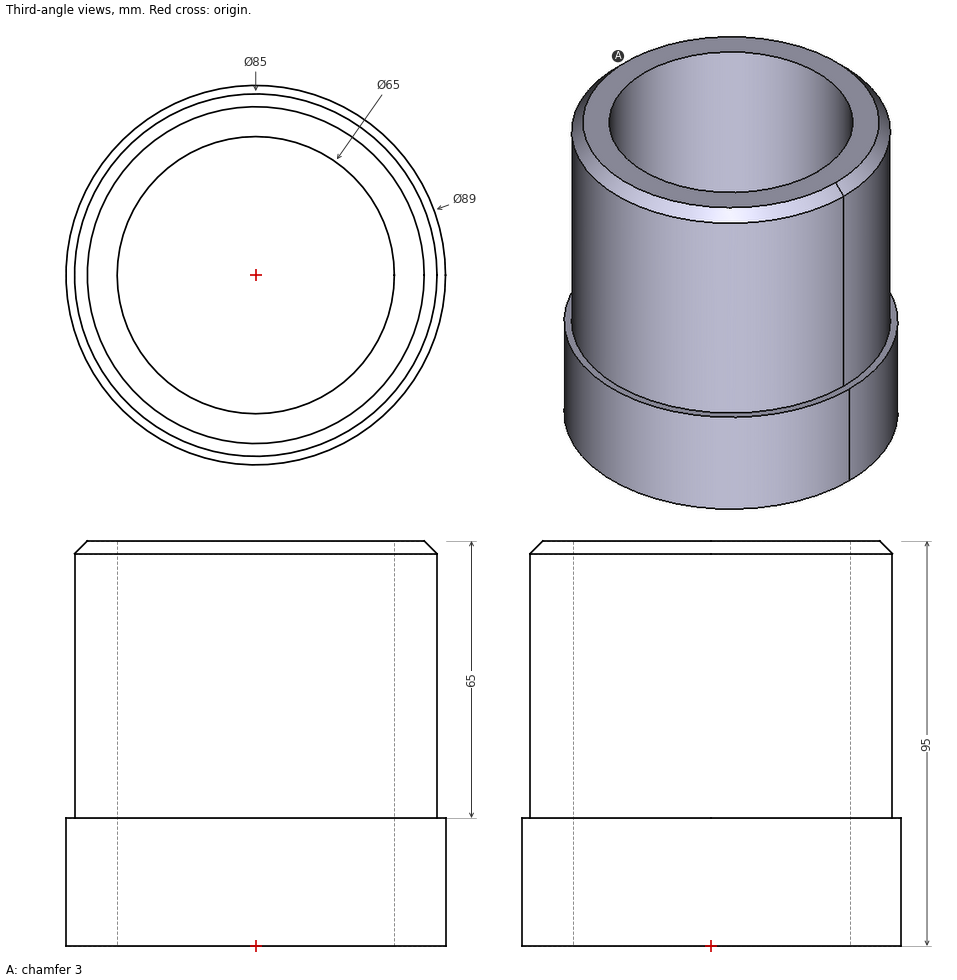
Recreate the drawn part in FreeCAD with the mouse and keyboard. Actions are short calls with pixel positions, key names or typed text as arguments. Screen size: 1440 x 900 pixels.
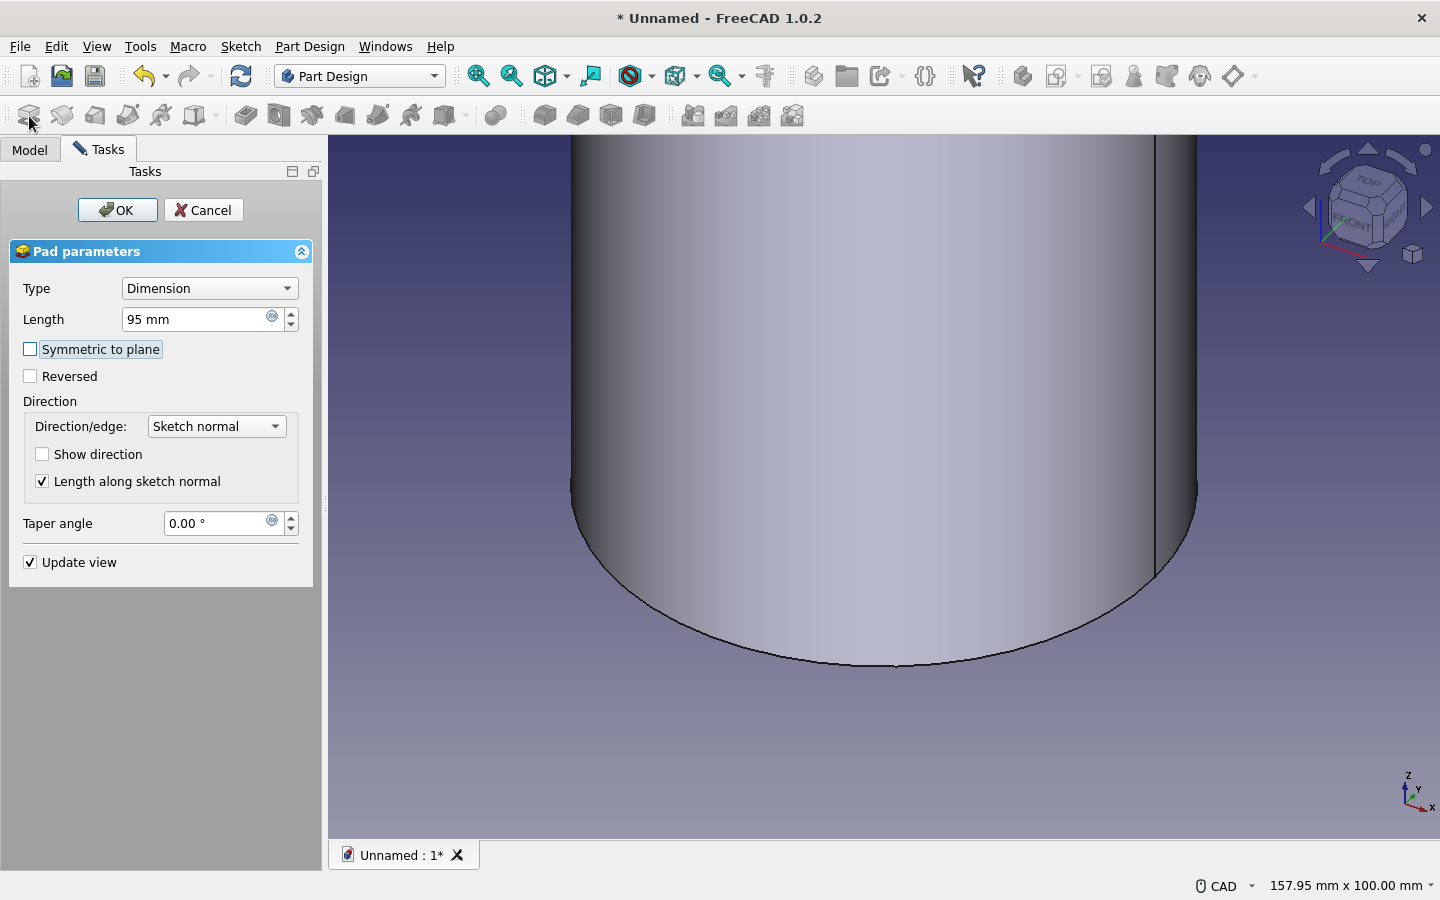
click(118, 210)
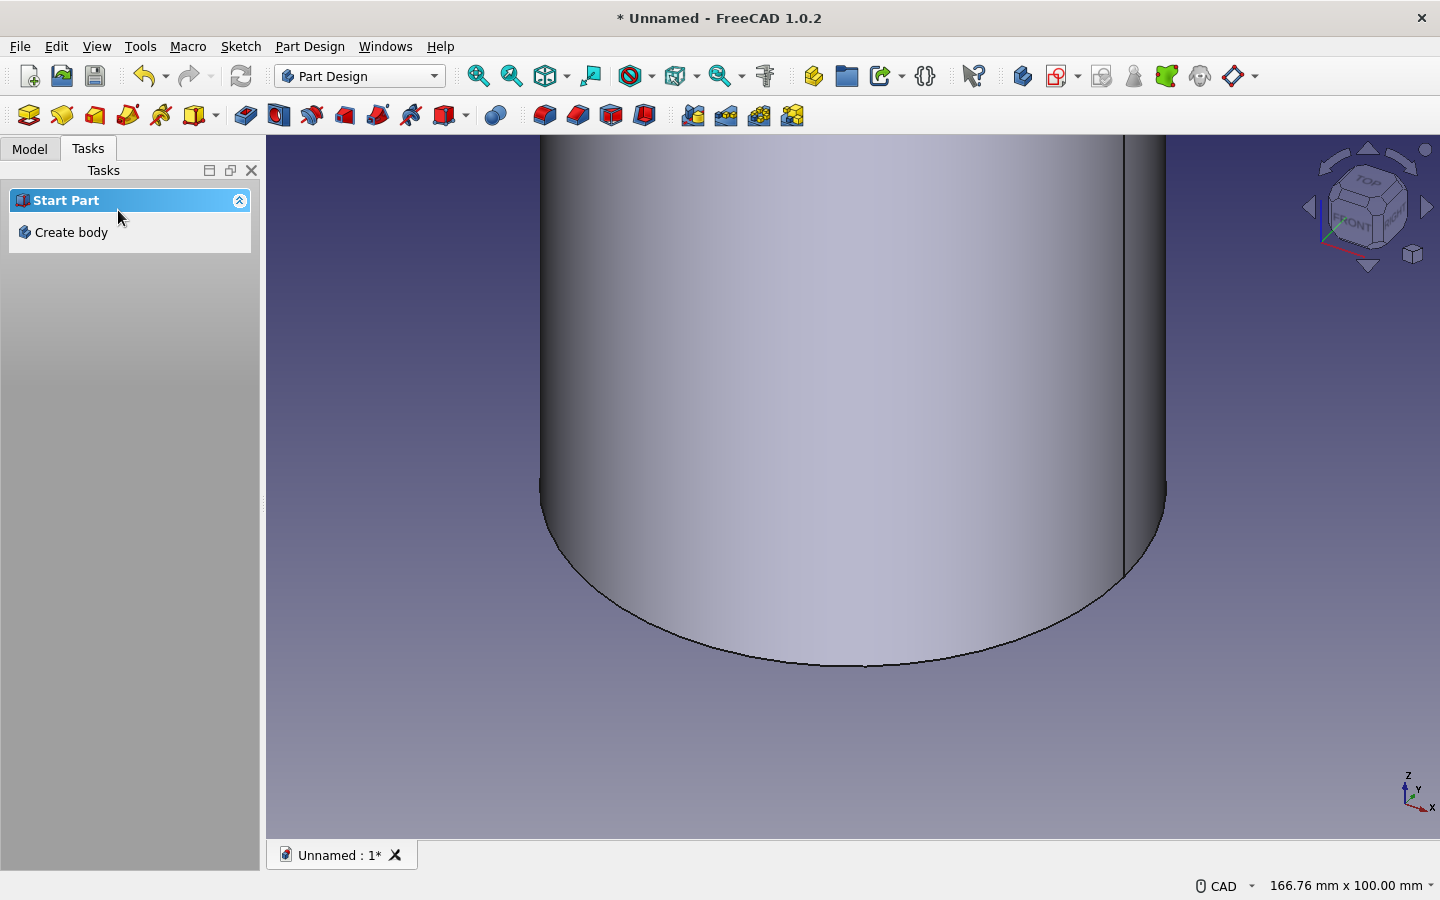
click(479, 76)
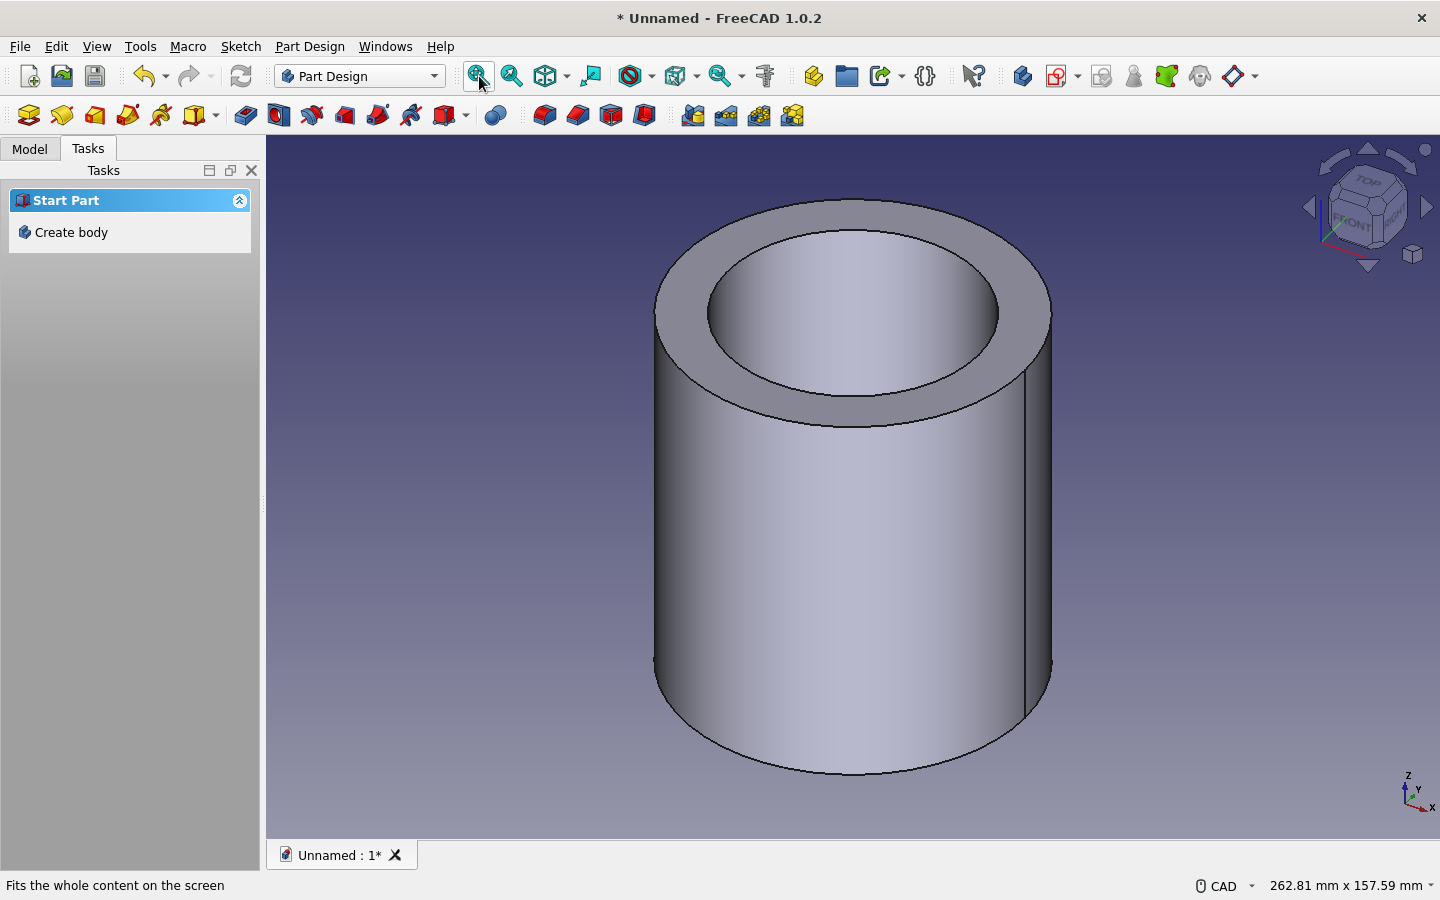
click(30, 148)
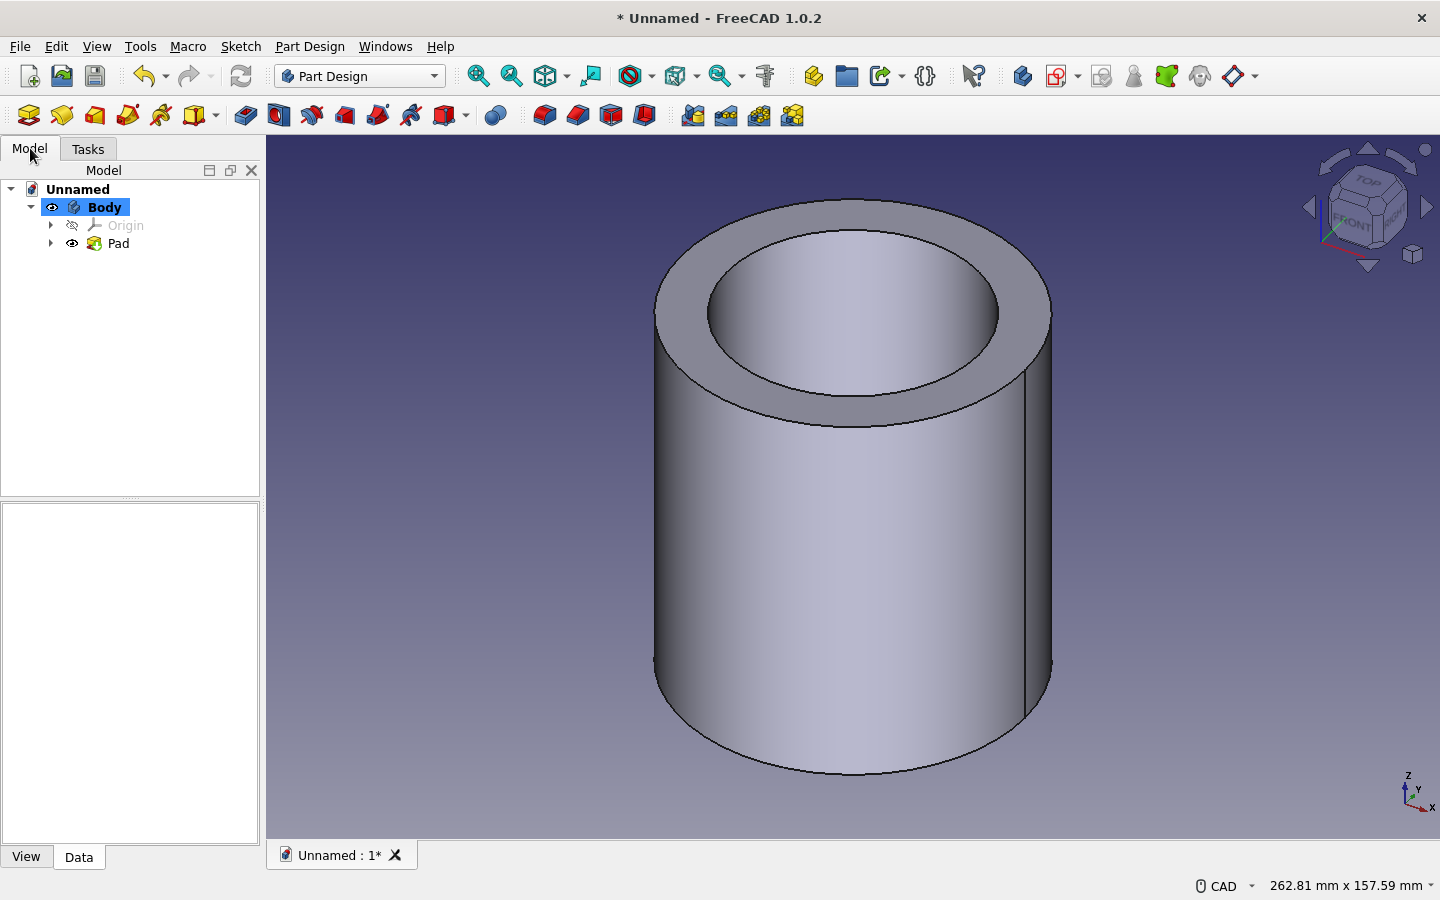
click(51, 225)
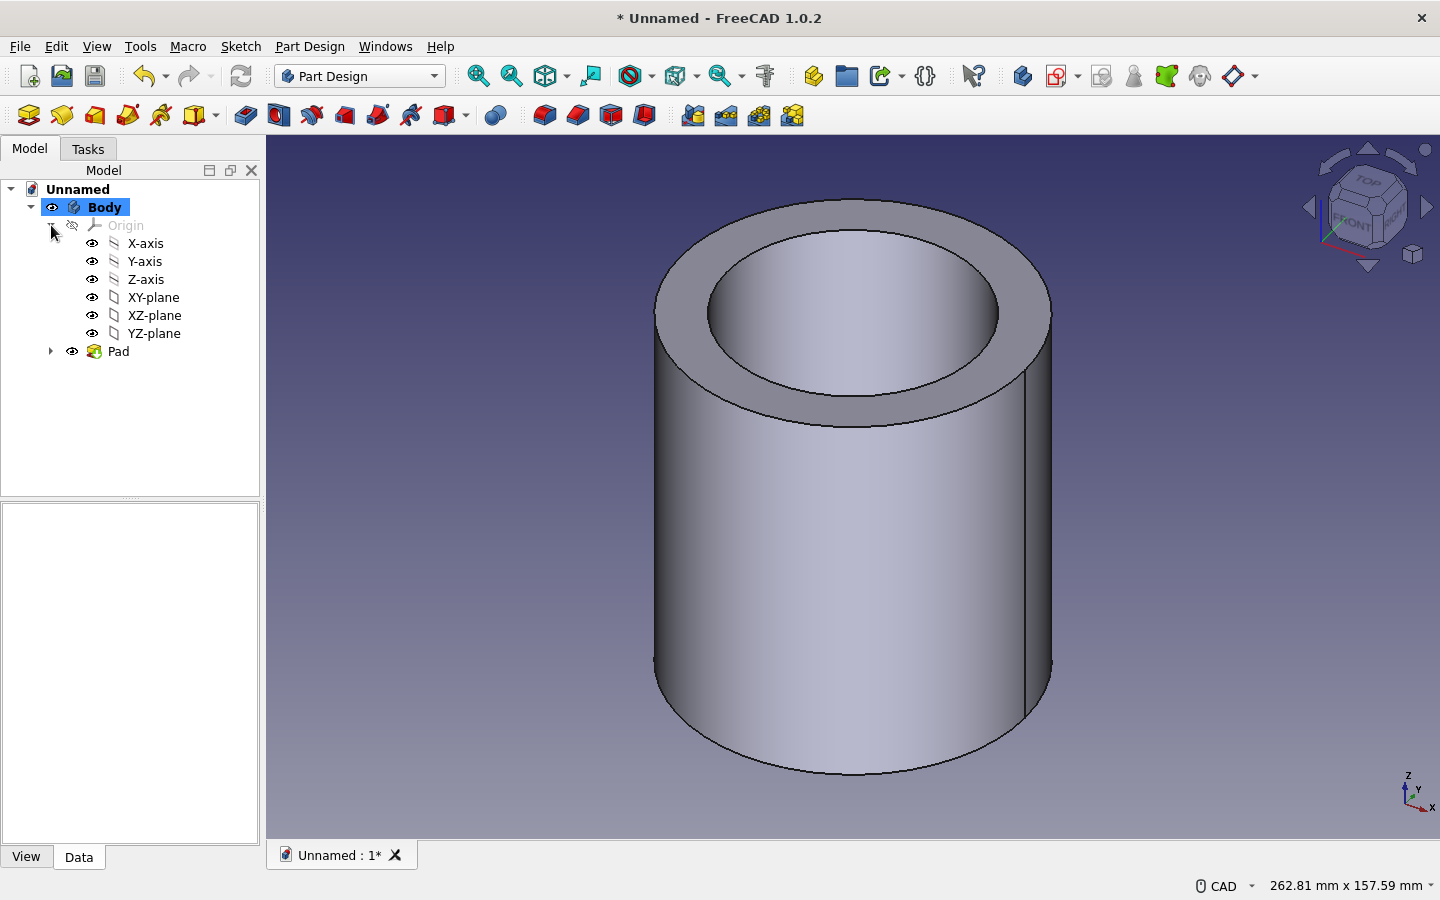
click(137, 297)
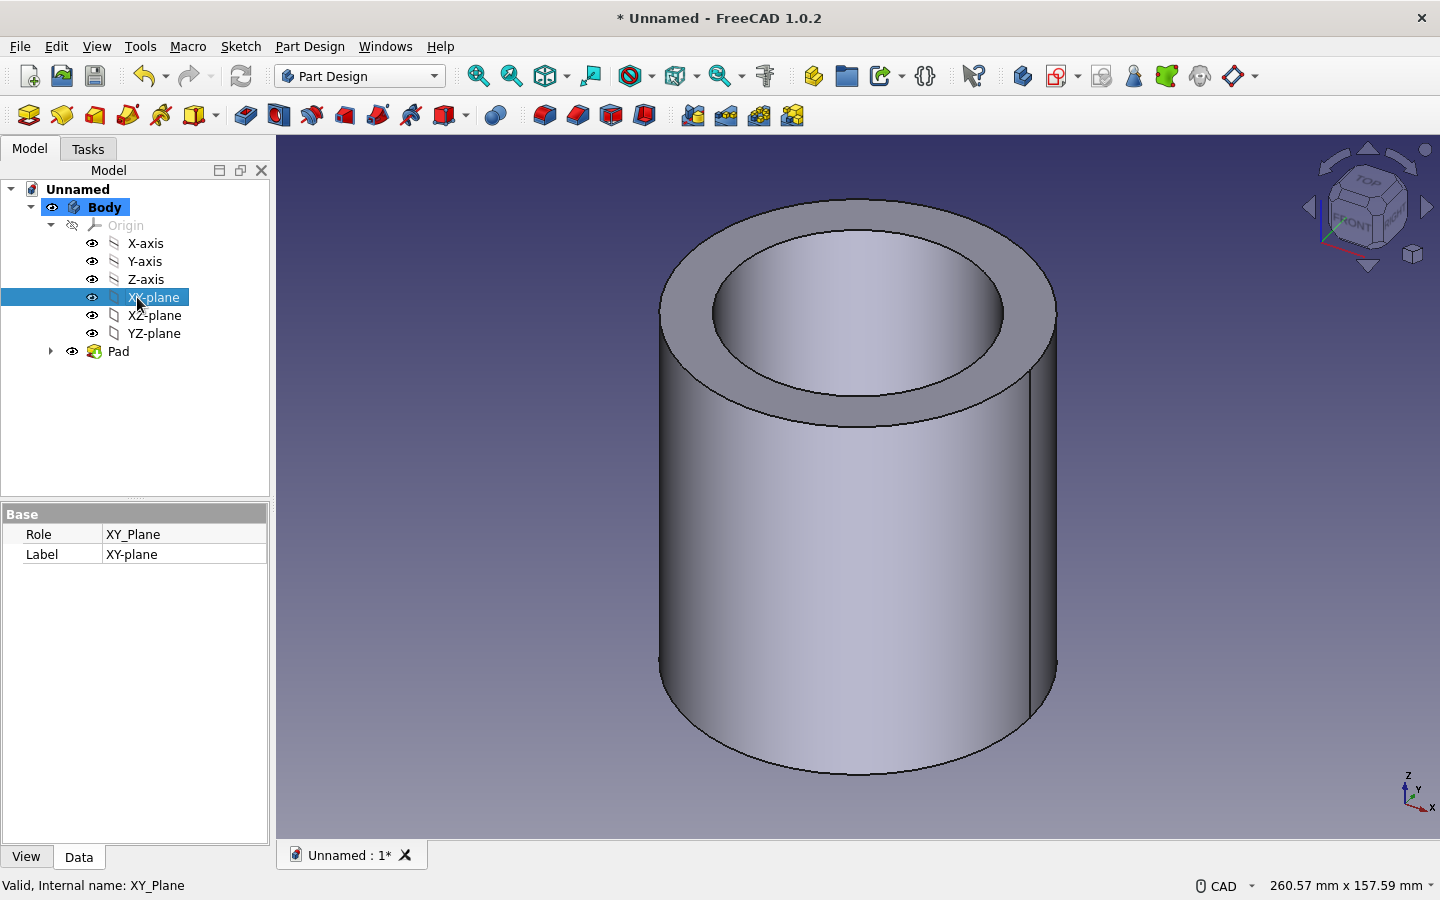
click(1232, 76)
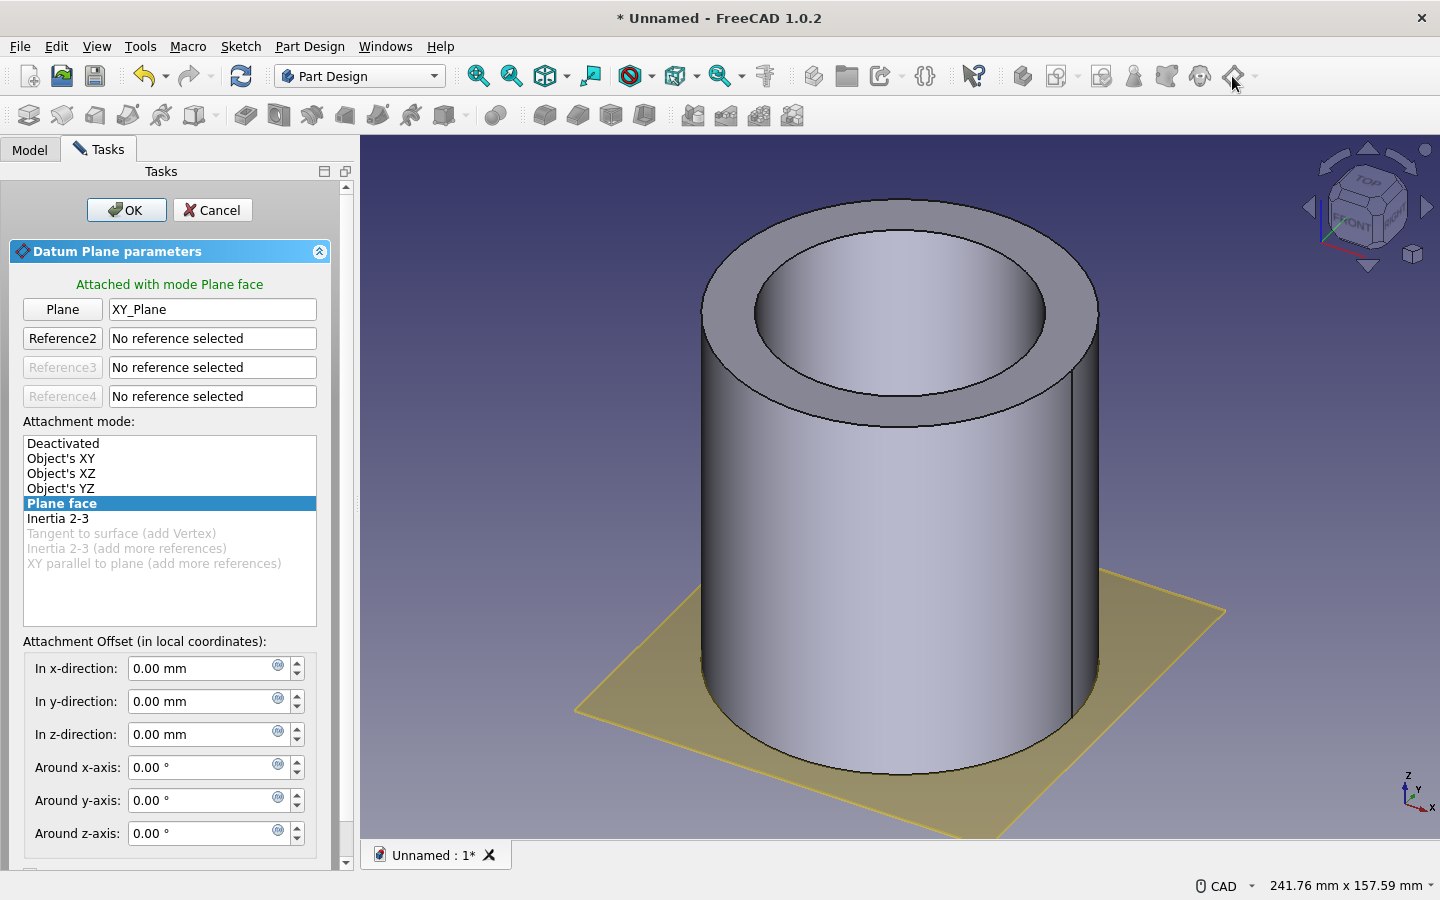
triple_click(210, 734)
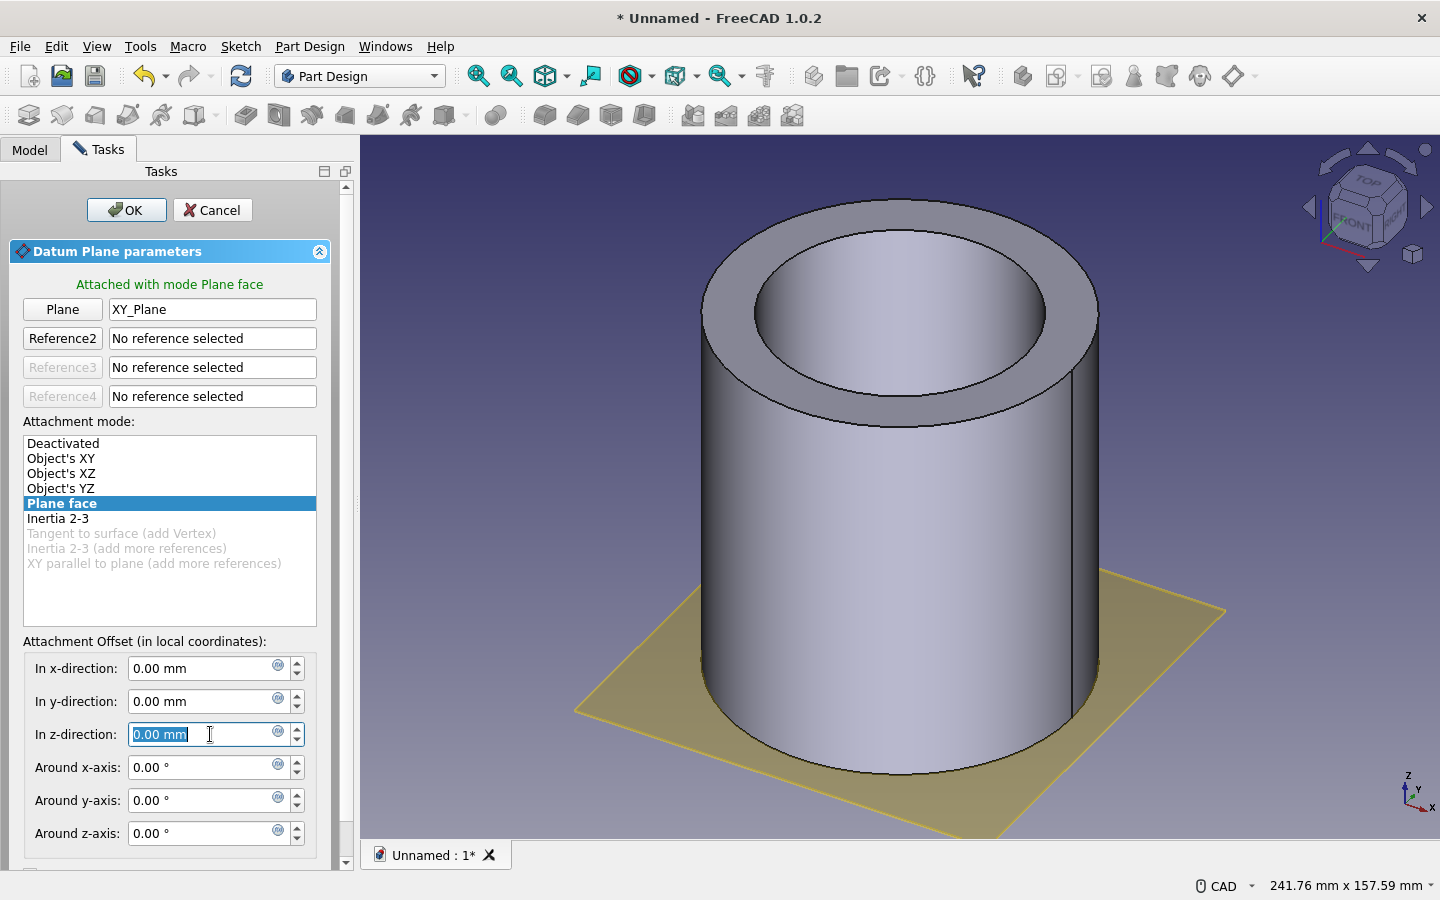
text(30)
key(Tab)